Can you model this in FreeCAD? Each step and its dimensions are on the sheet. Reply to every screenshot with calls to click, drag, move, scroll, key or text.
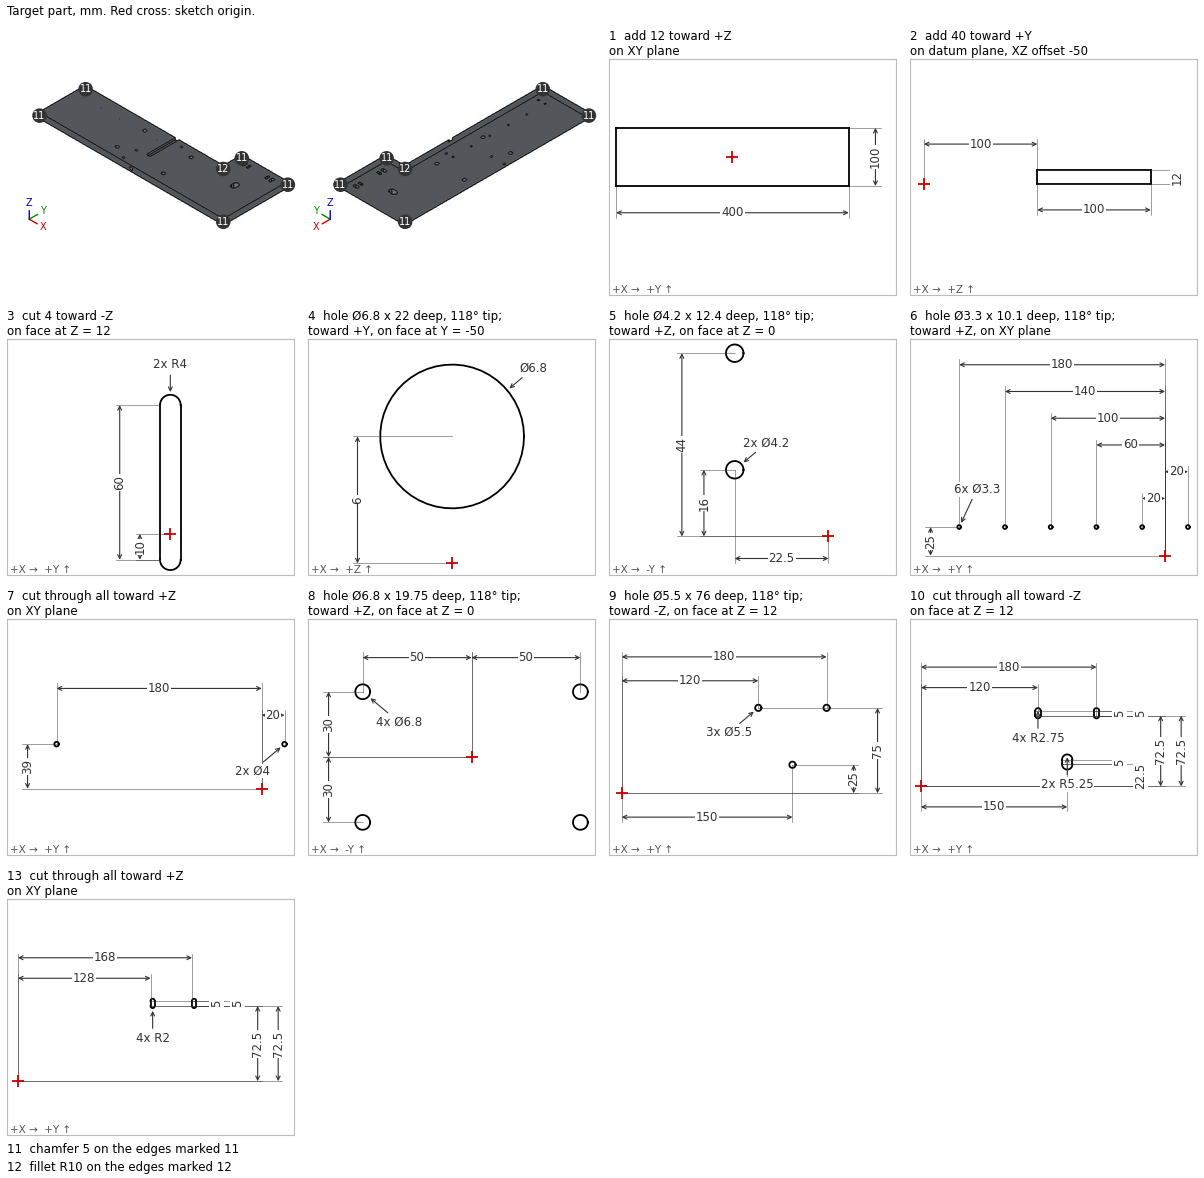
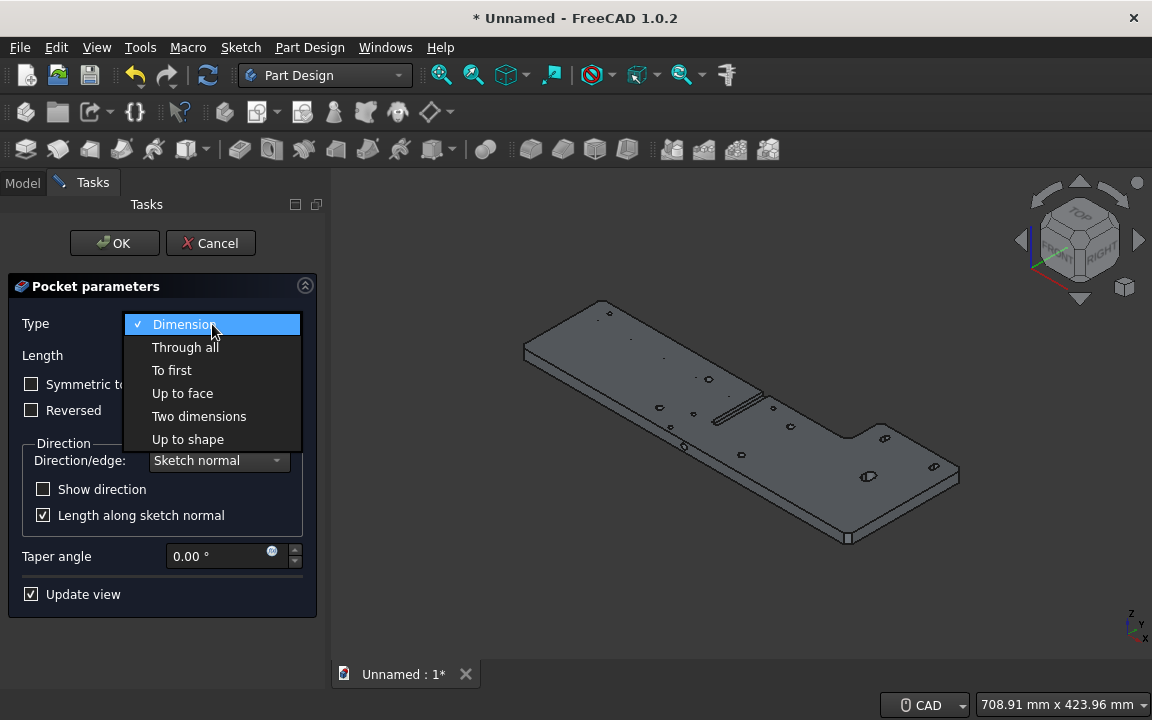
click(212, 348)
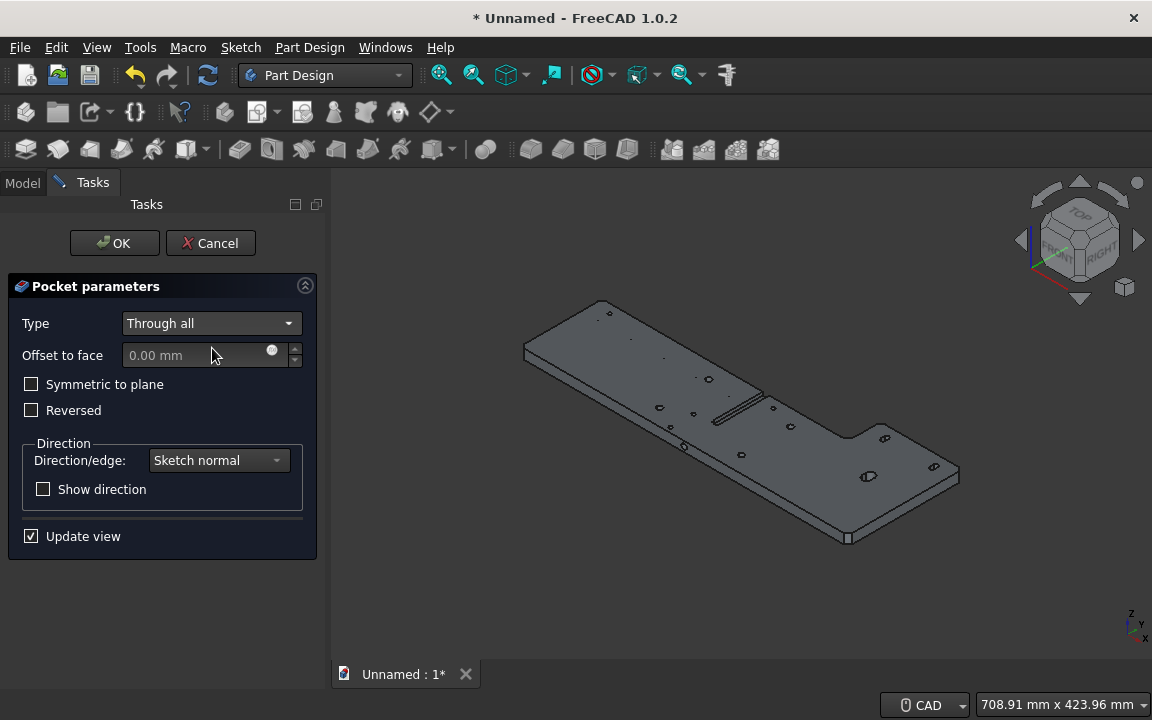
click(30, 410)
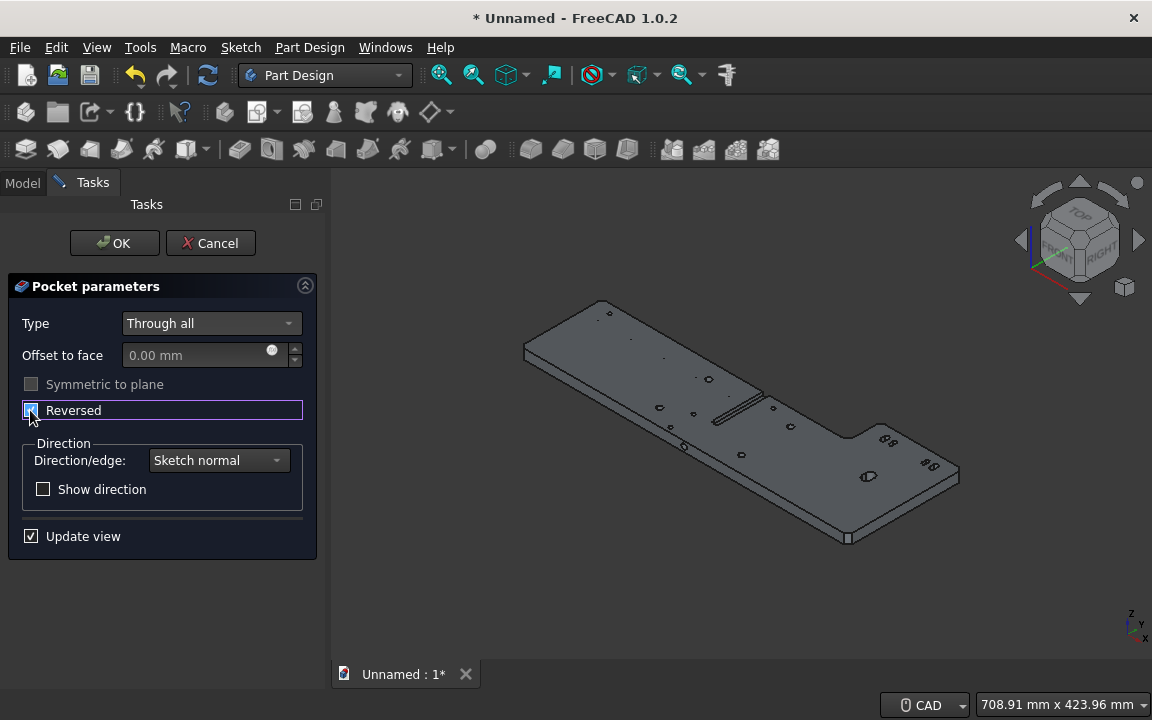
click(115, 243)